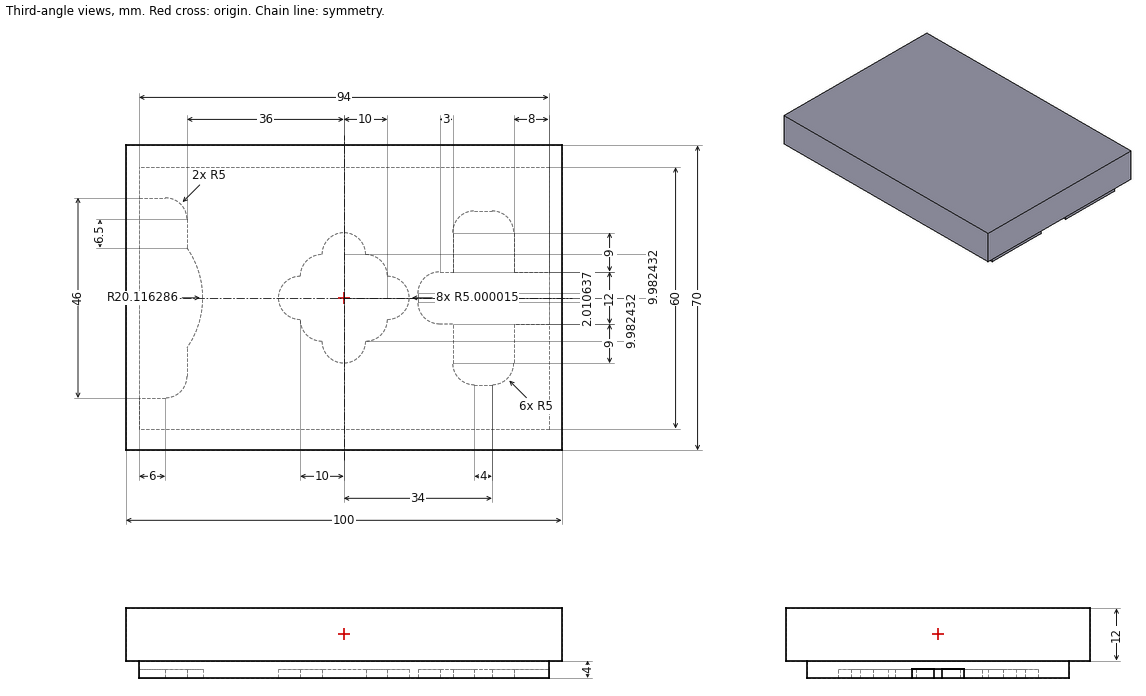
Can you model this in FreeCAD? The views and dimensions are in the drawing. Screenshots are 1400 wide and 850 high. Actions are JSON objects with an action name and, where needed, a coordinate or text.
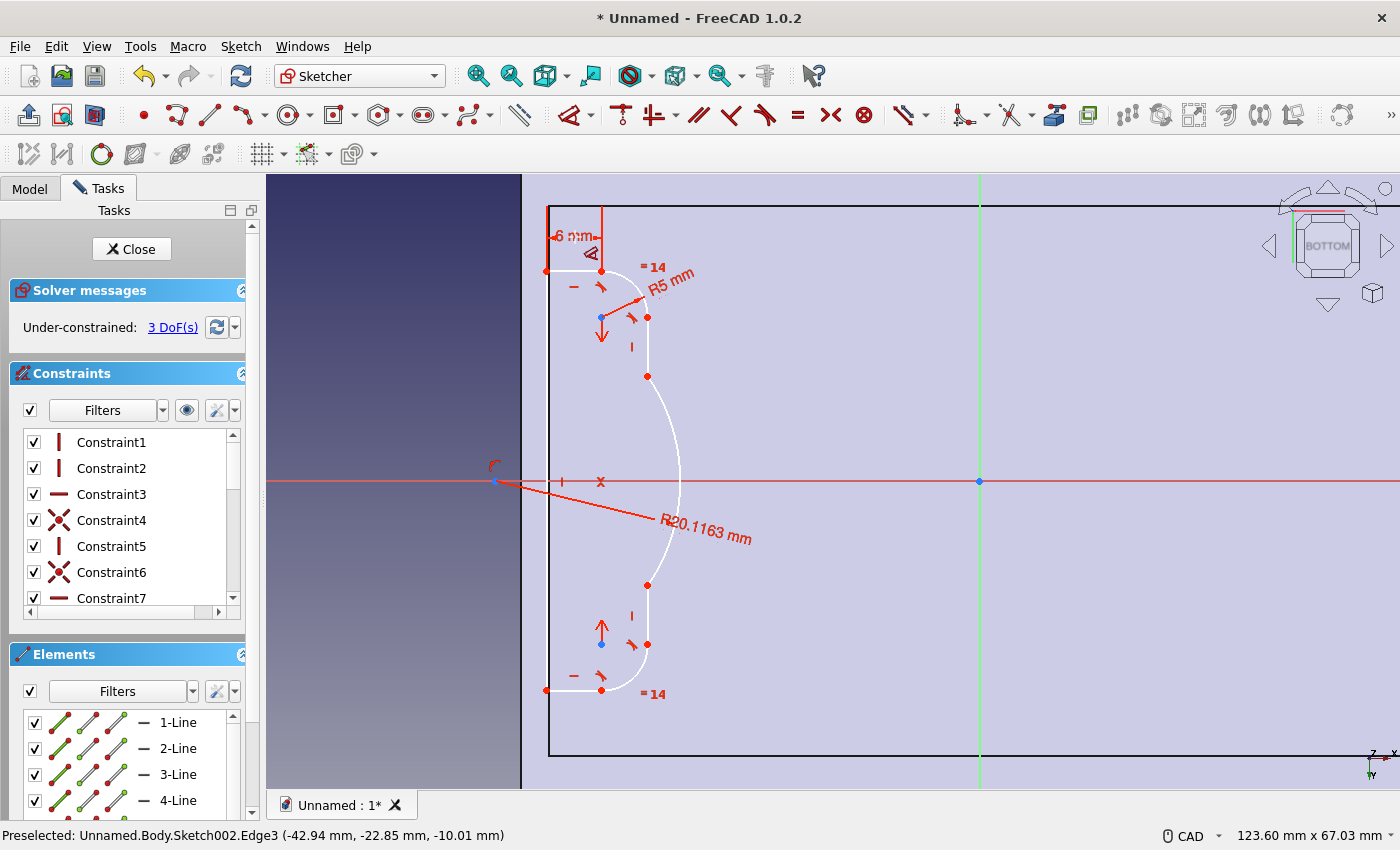
{"action": "left_click", "coordinate": [547, 397]}
{"action": "left_click", "coordinate": [513, 385]}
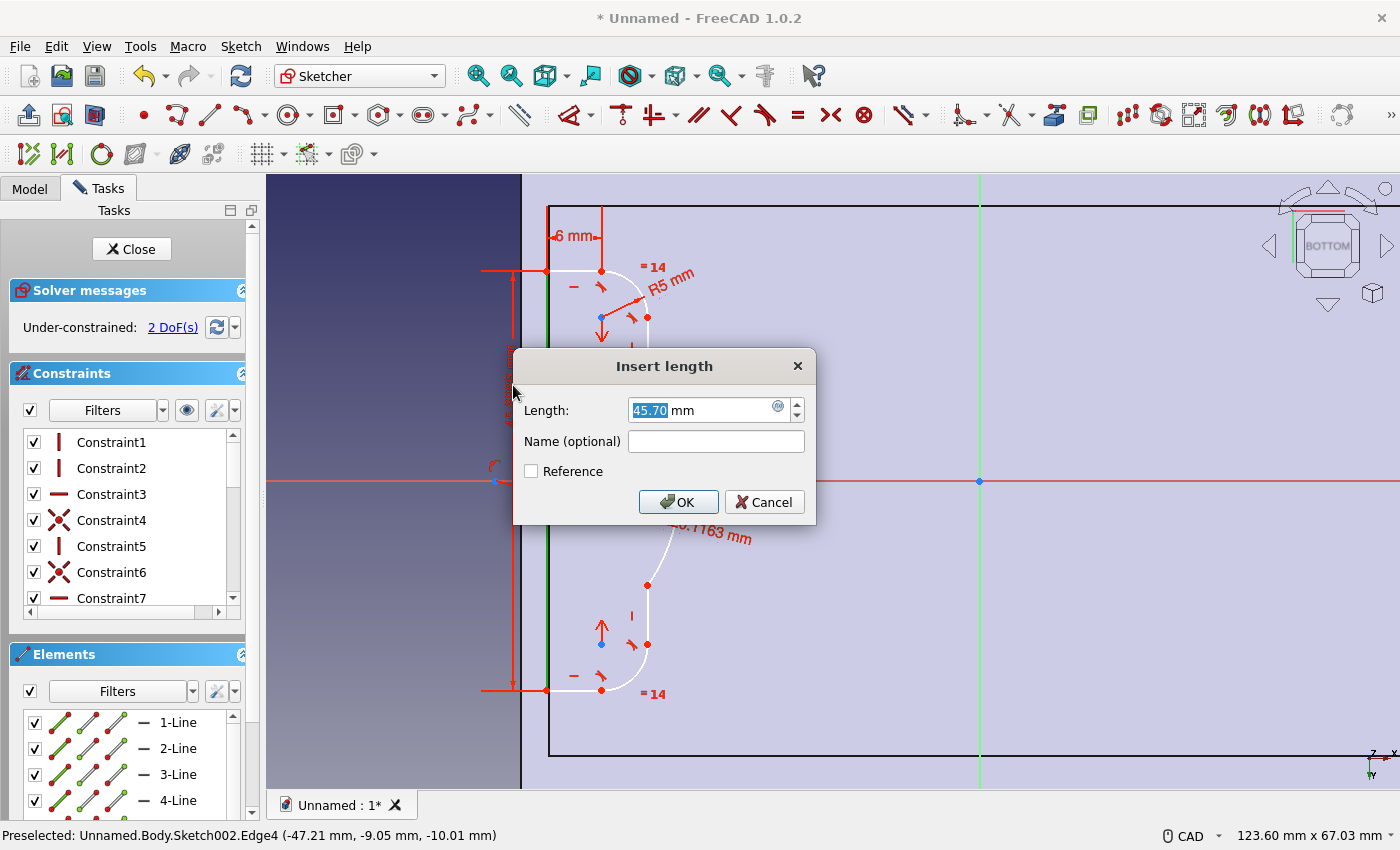
{"action": "type", "text": "46"}
{"action": "key", "text": "Return"}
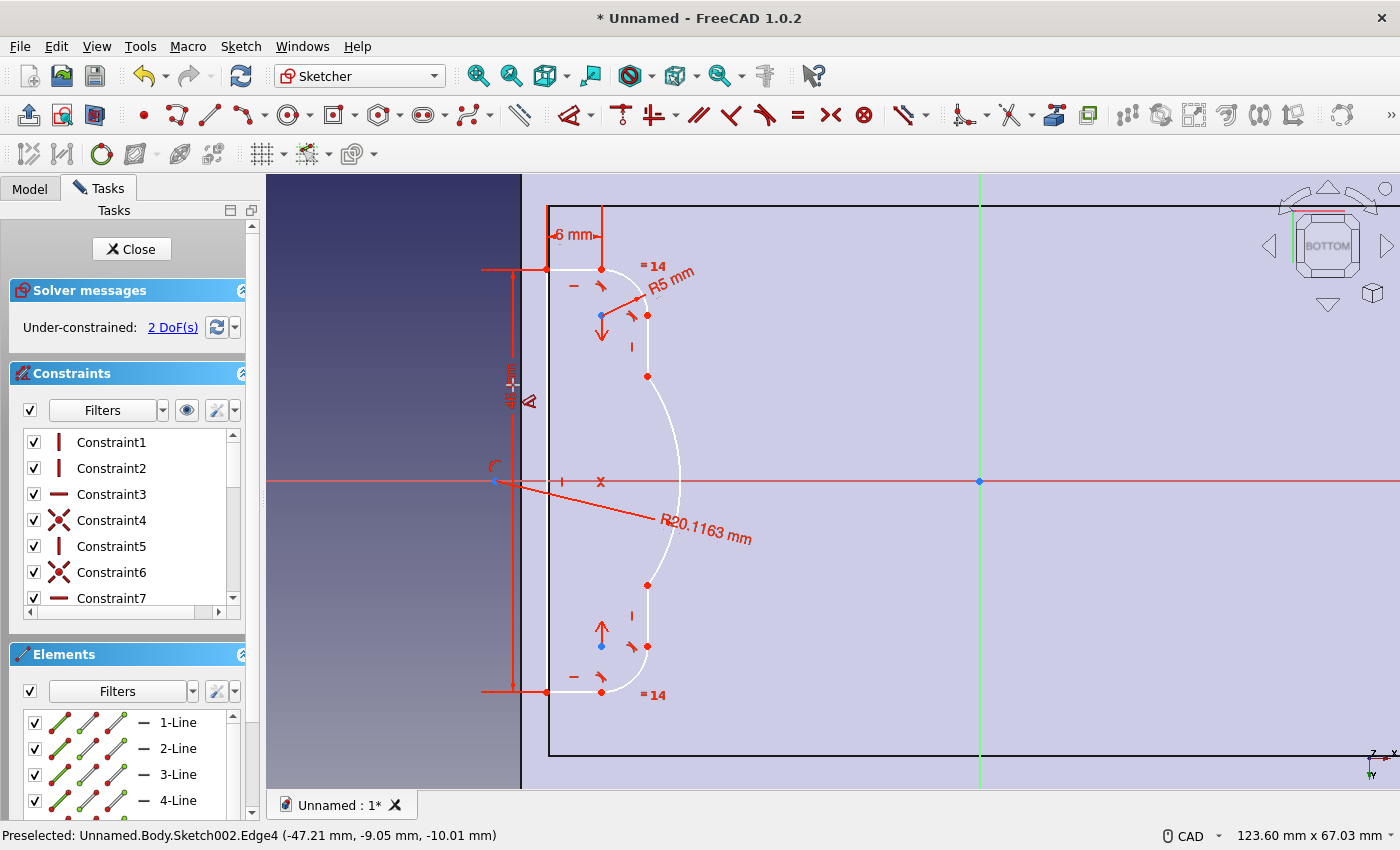
{"action": "left_click", "coordinate": [648, 628]}
{"action": "left_click", "coordinate": [614, 616]}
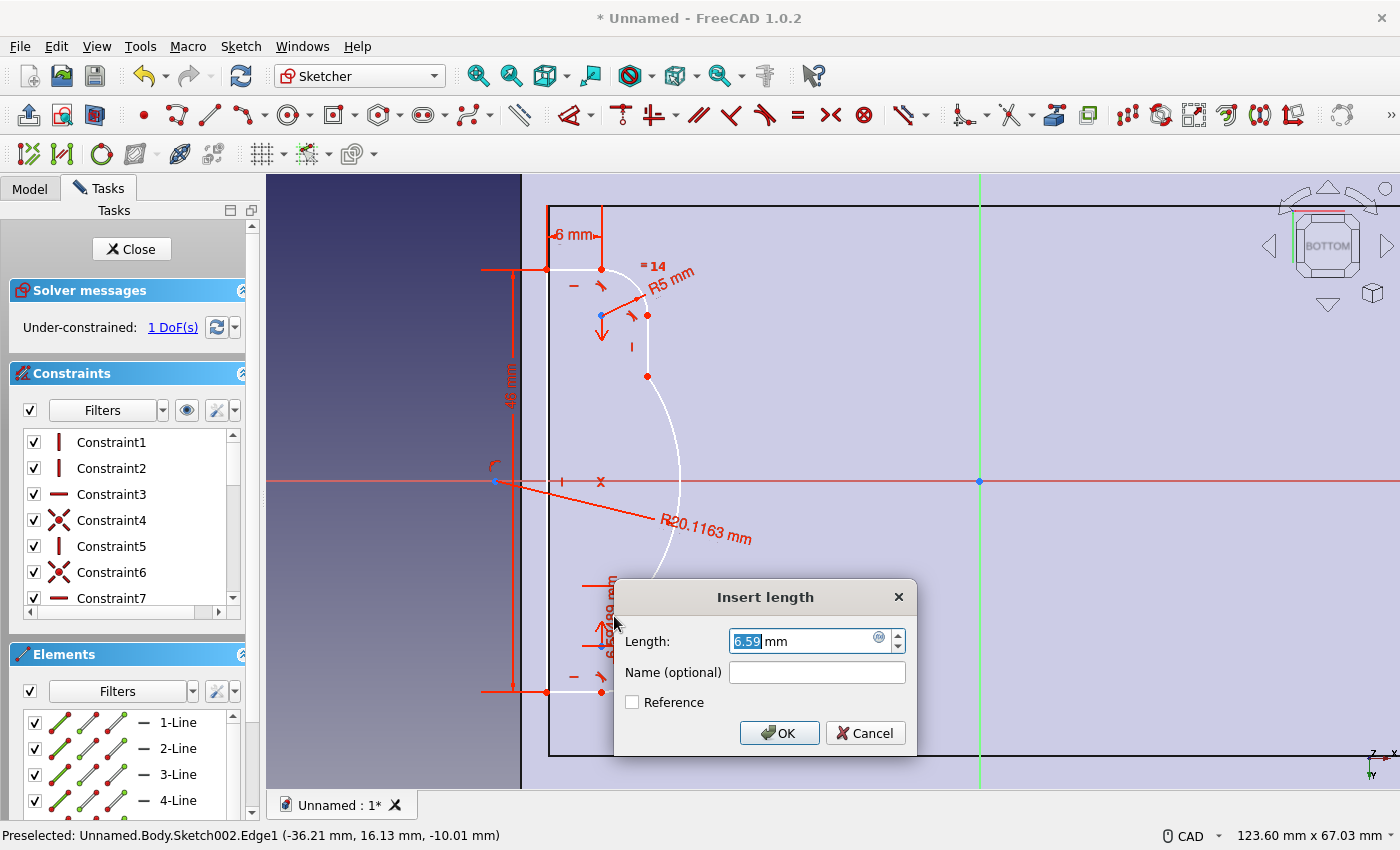
{"action": "type", "text": "6.5"}
{"action": "key", "text": "Return"}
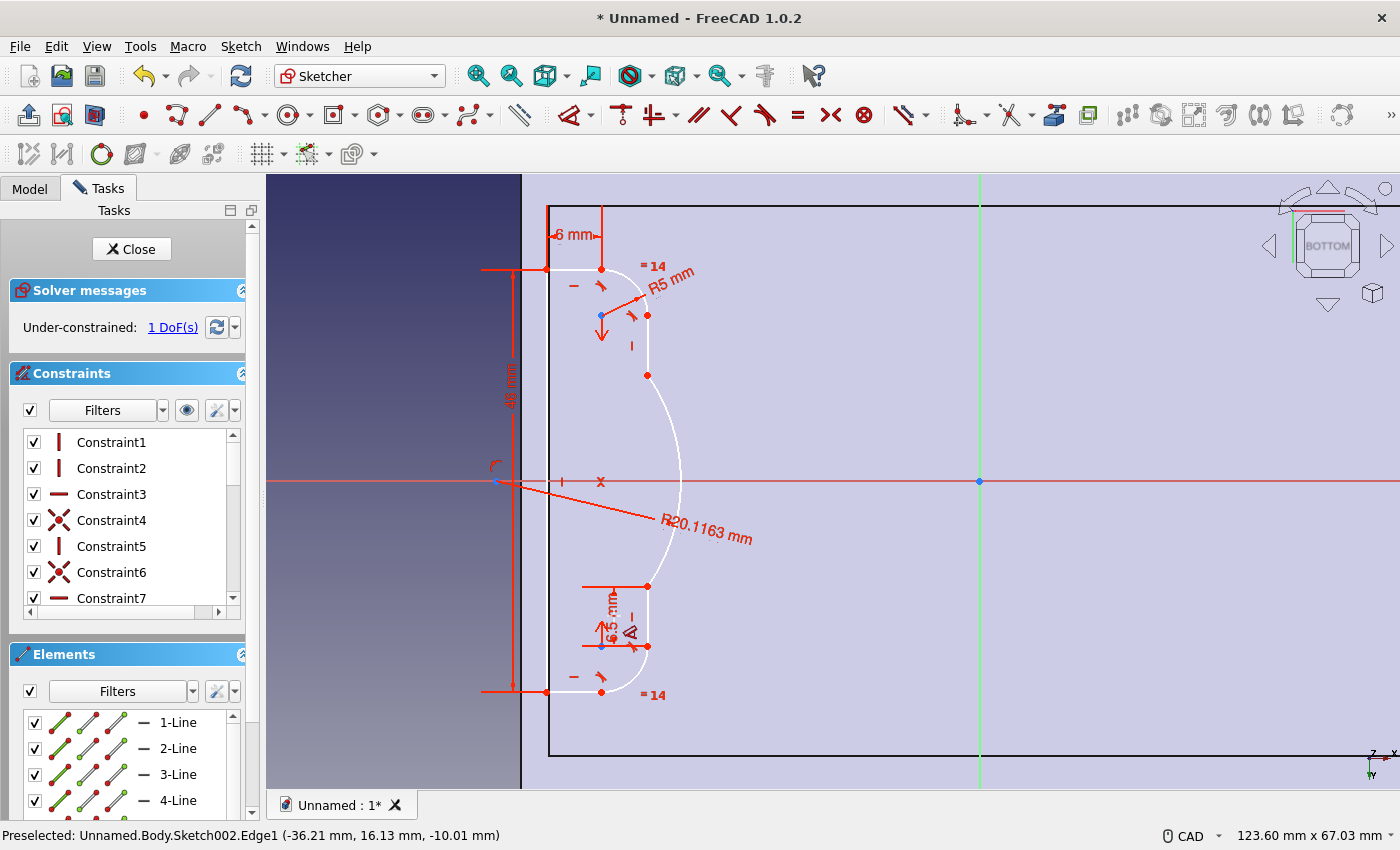
{"action": "left_click", "coordinate": [648, 646]}
{"action": "left_click", "coordinate": [814, 680]}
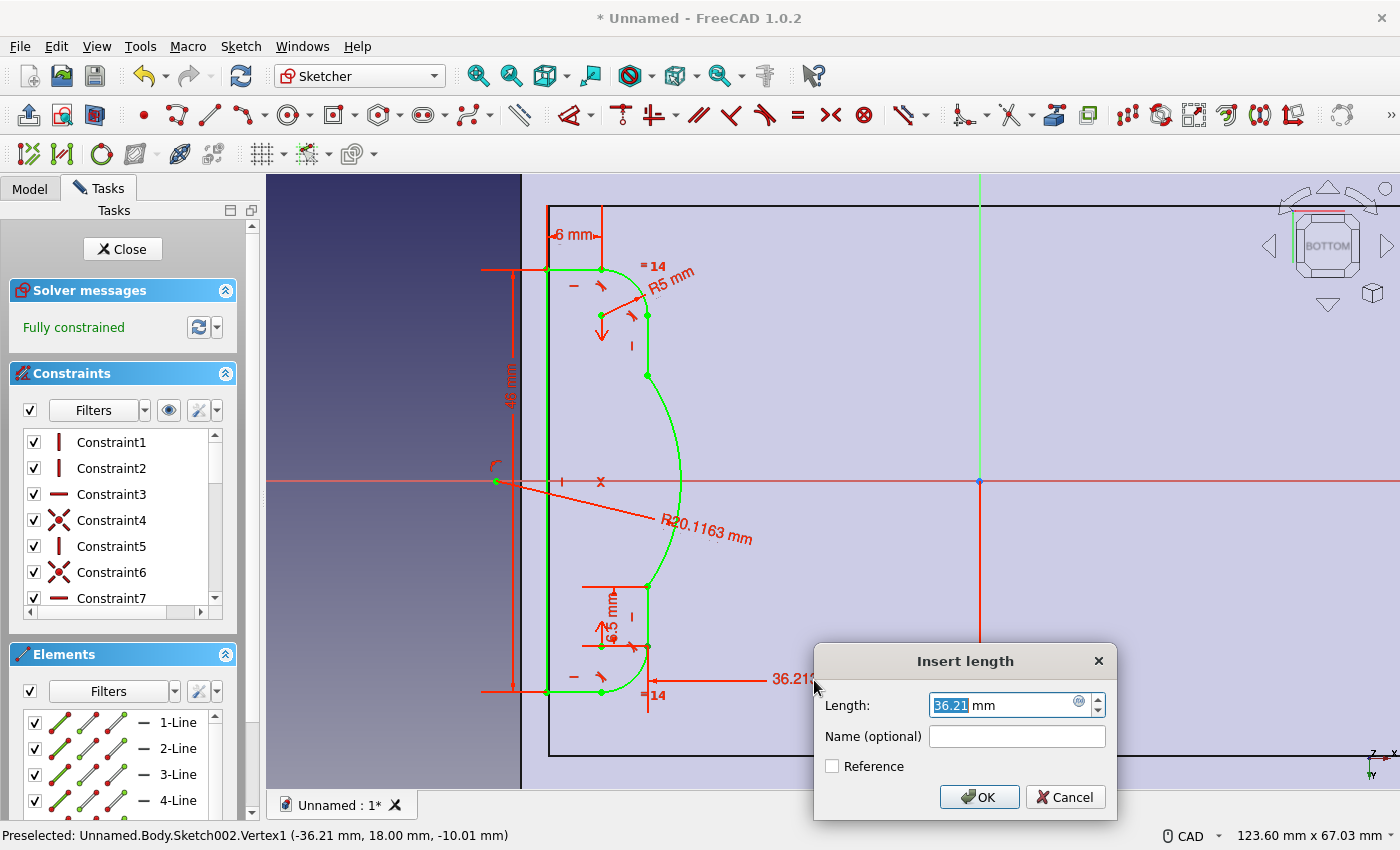
{"action": "type", "text": "36"}
{"action": "key", "text": "Return"}
{"action": "key", "text": "Escape"}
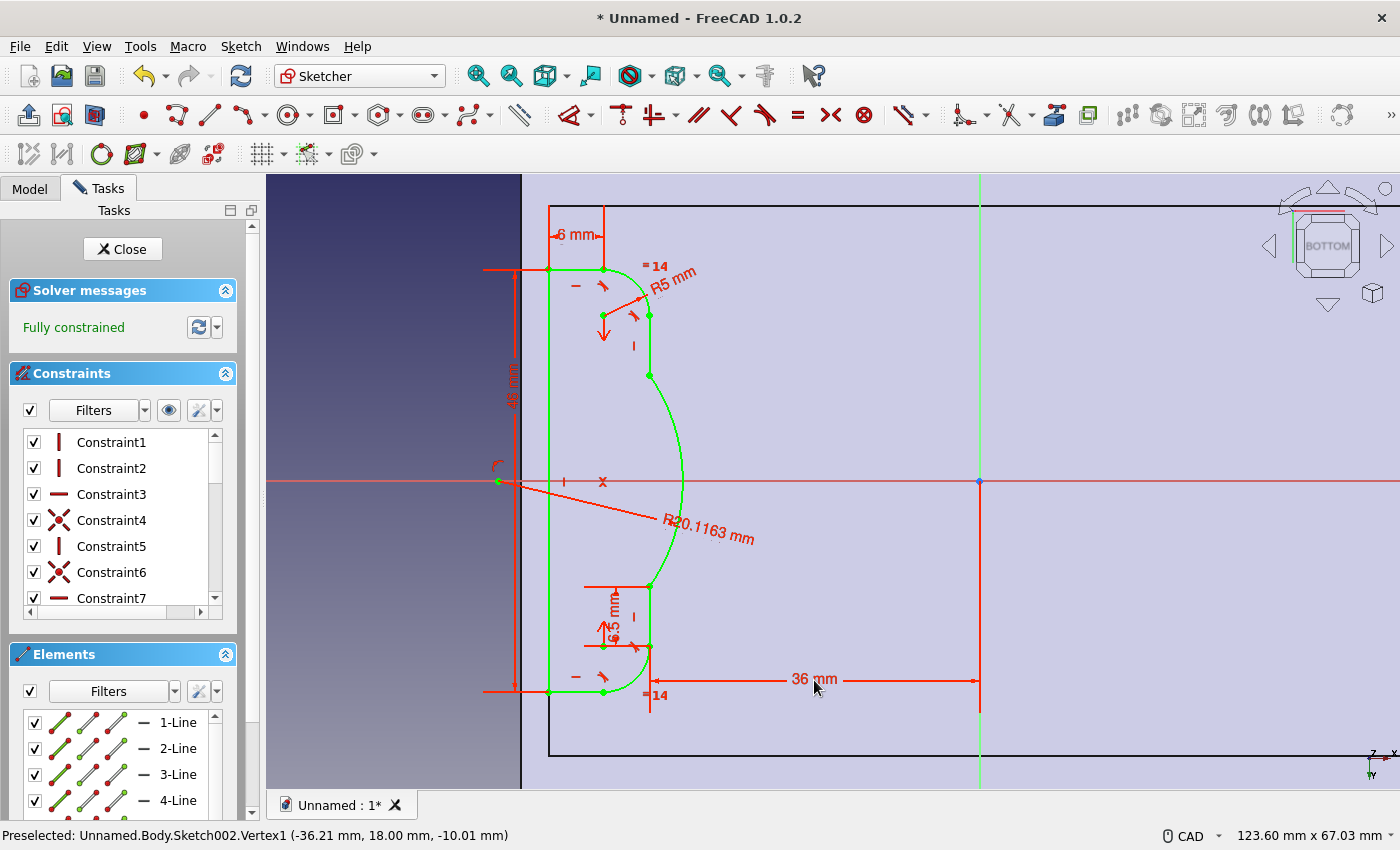
{"action": "left_click", "coordinate": [123, 249]}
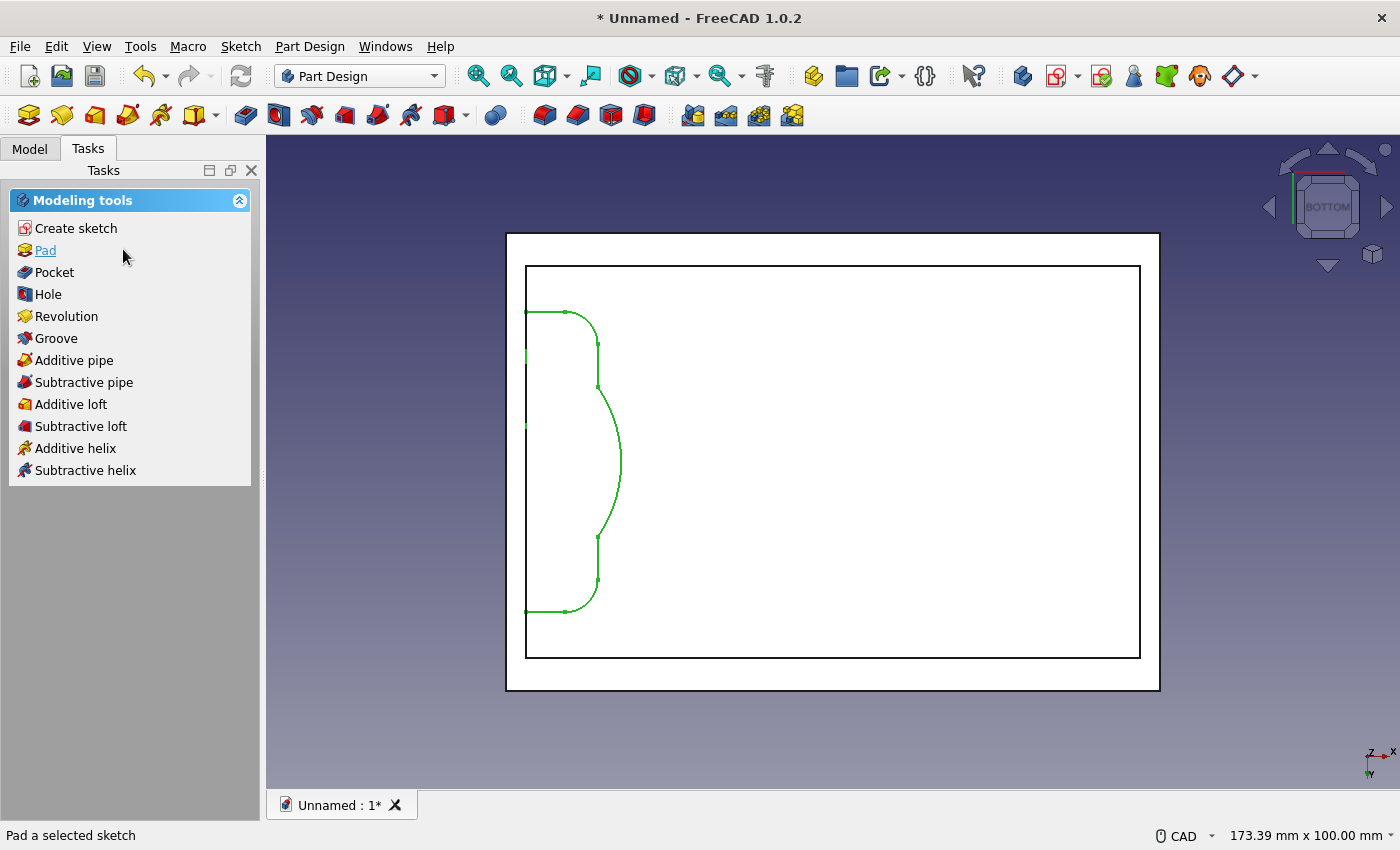
{"action": "left_click", "coordinate": [246, 116]}